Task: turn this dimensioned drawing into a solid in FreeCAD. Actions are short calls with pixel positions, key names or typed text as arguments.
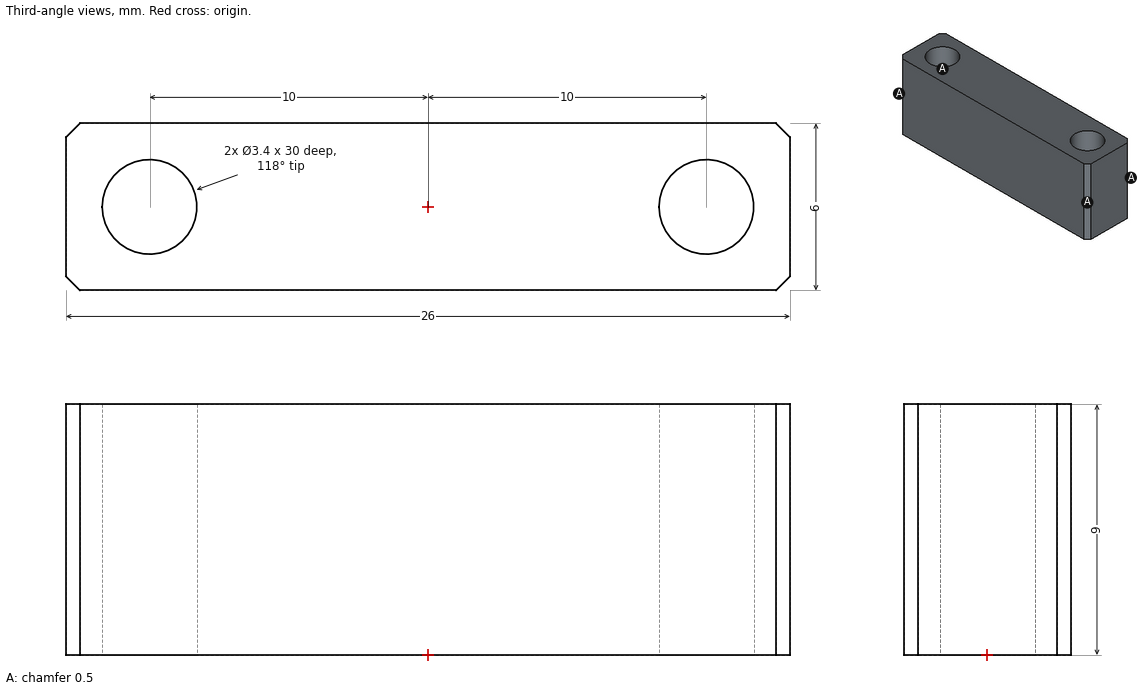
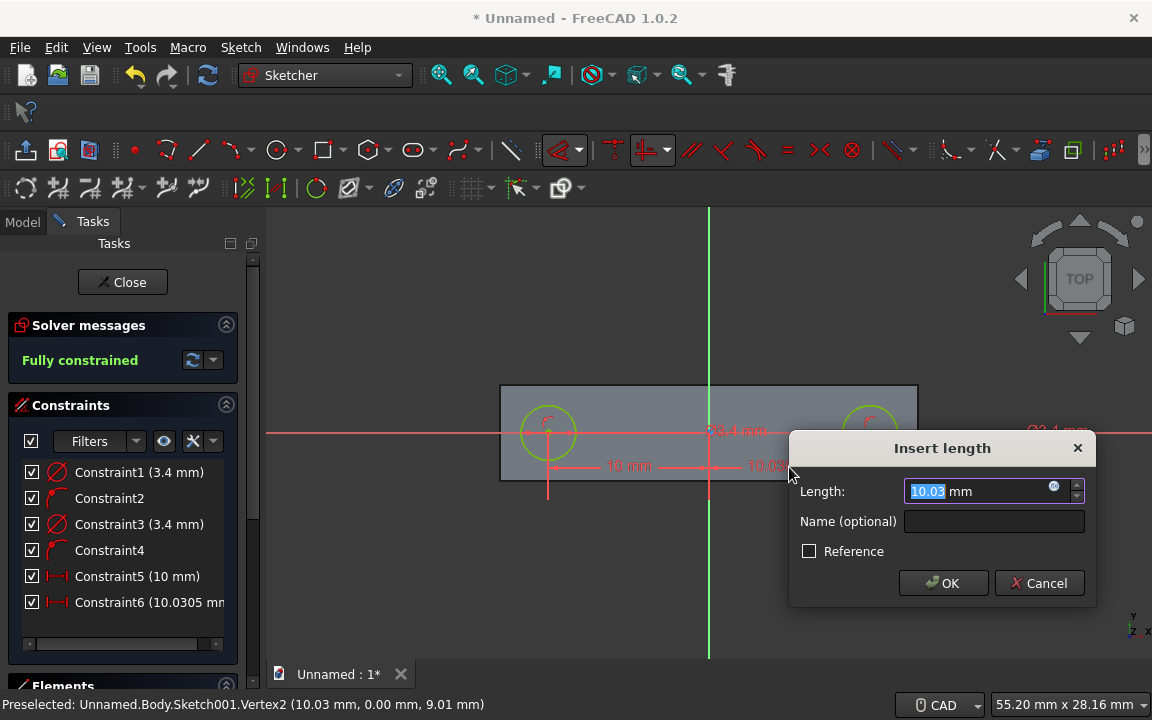
text(10)
key(Return)
key(Escape)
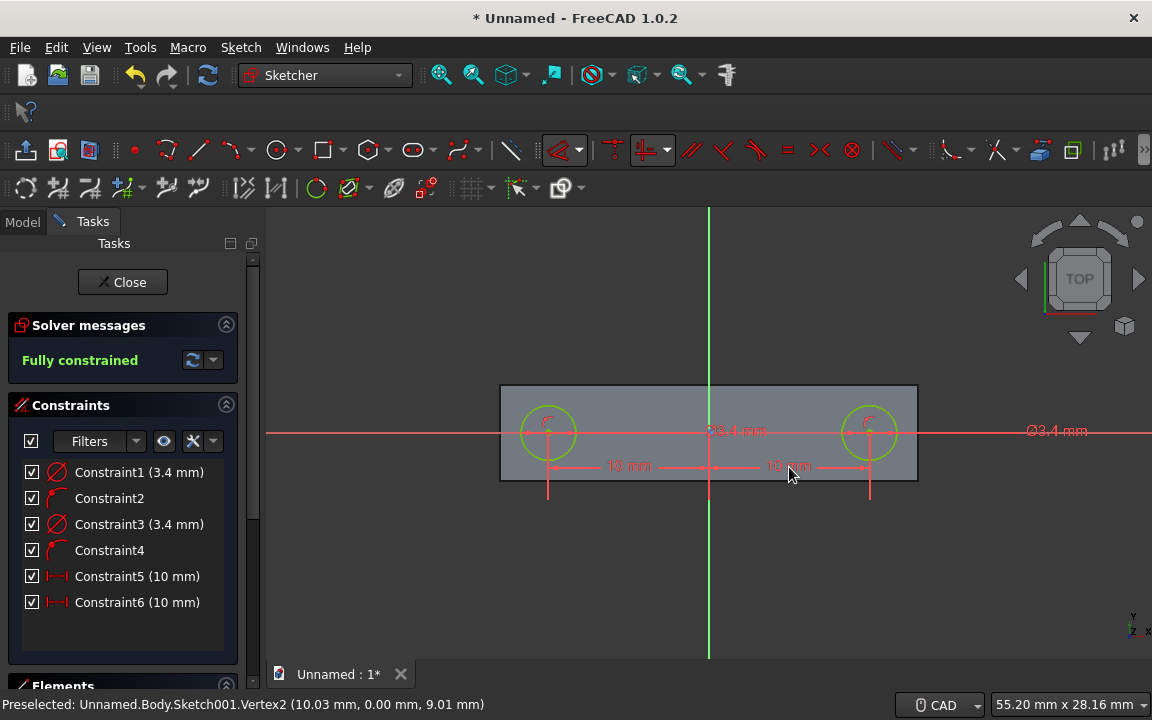
click(123, 282)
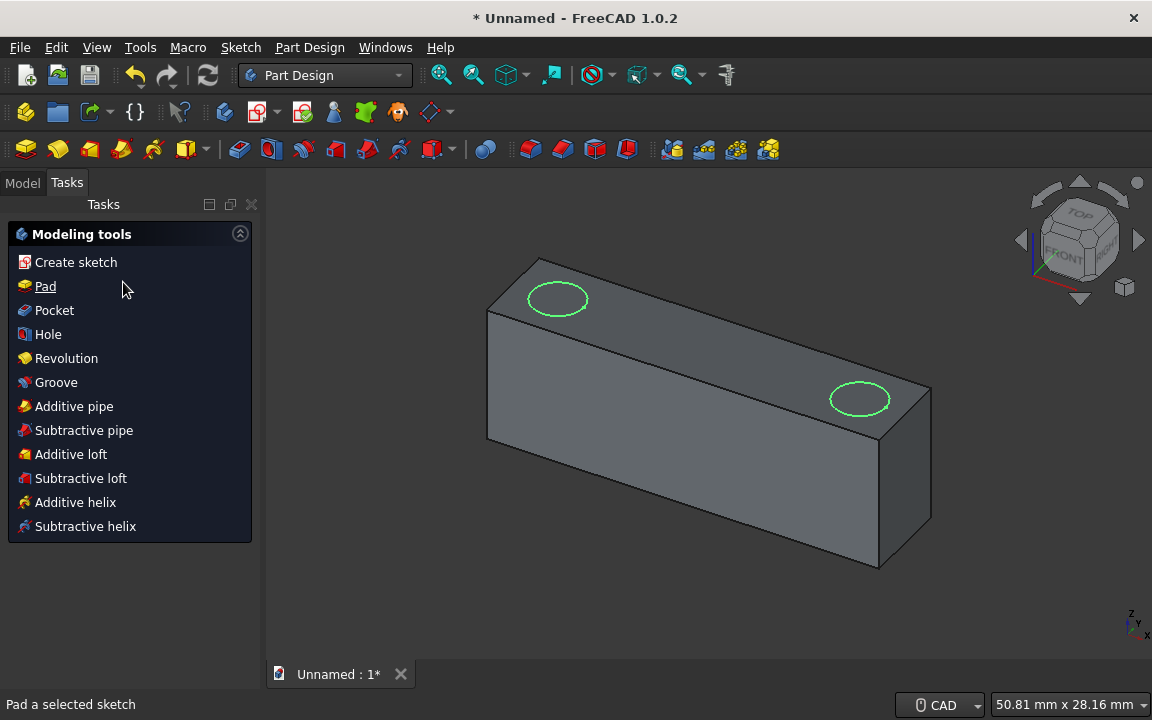
click(272, 150)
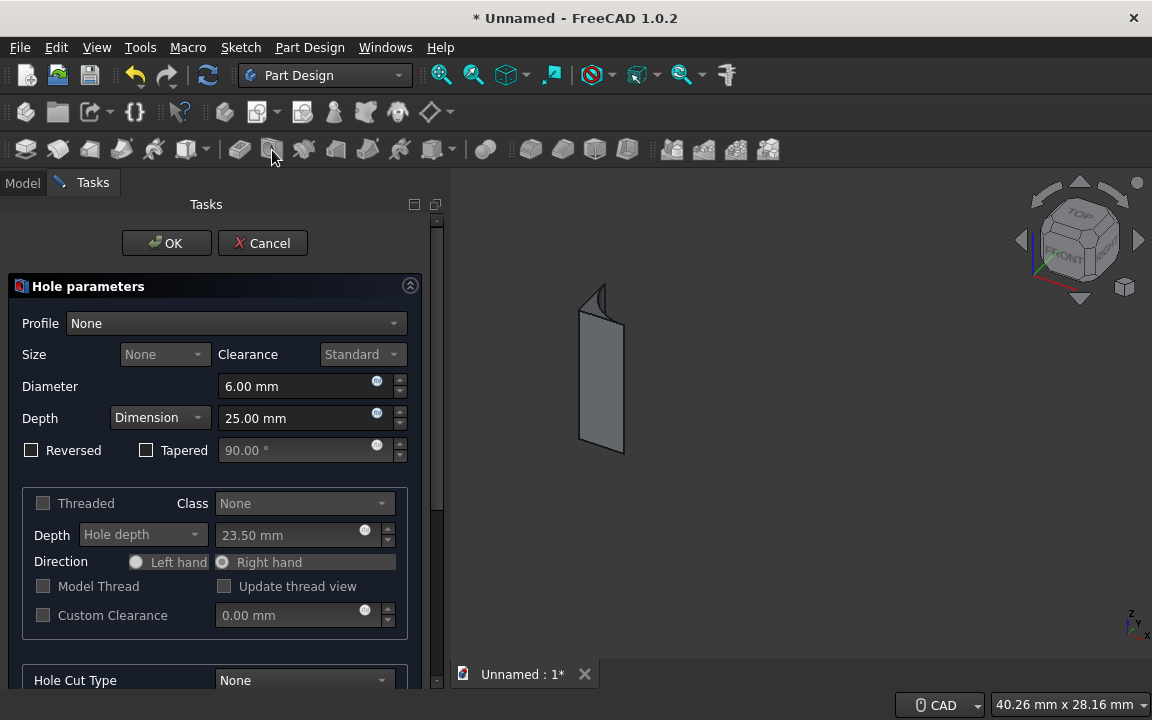
triple_click(305, 386)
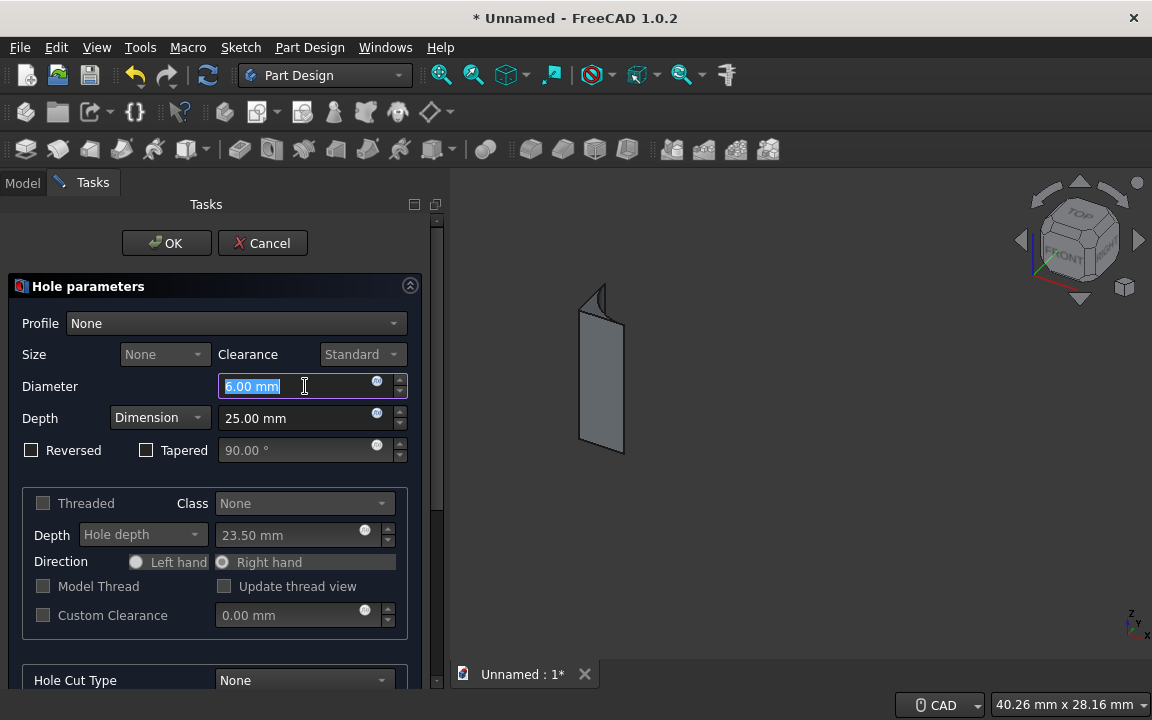
text(3.4)
key(Tab)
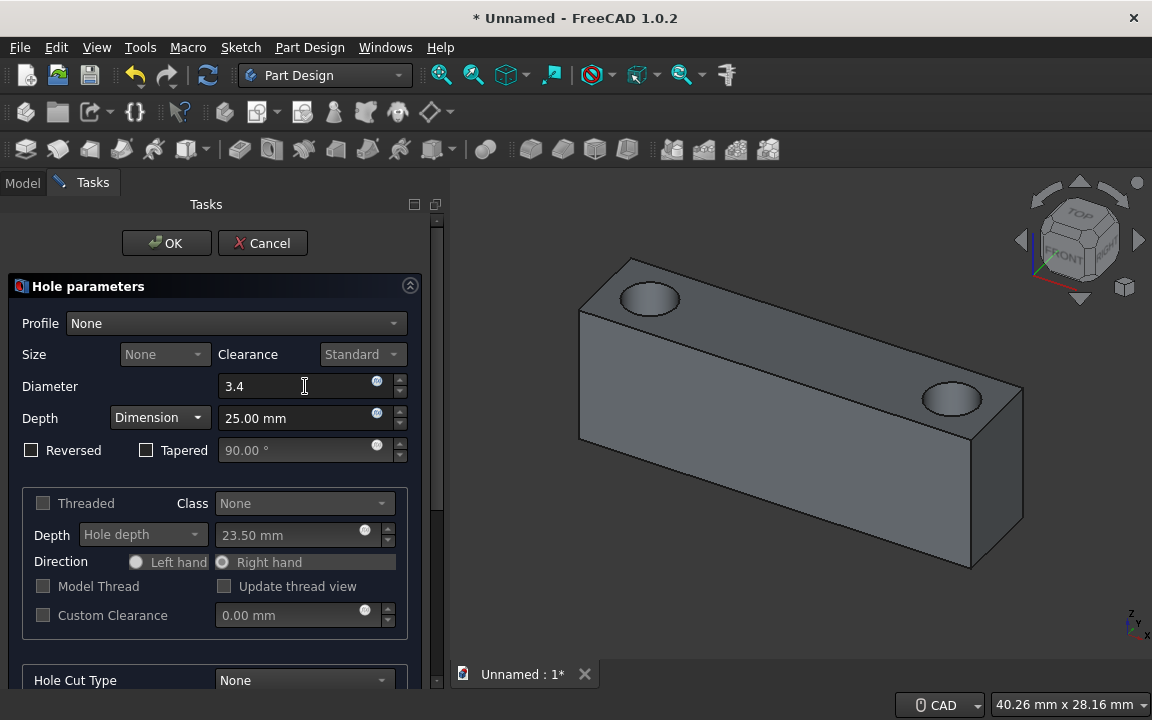
triple_click(305, 418)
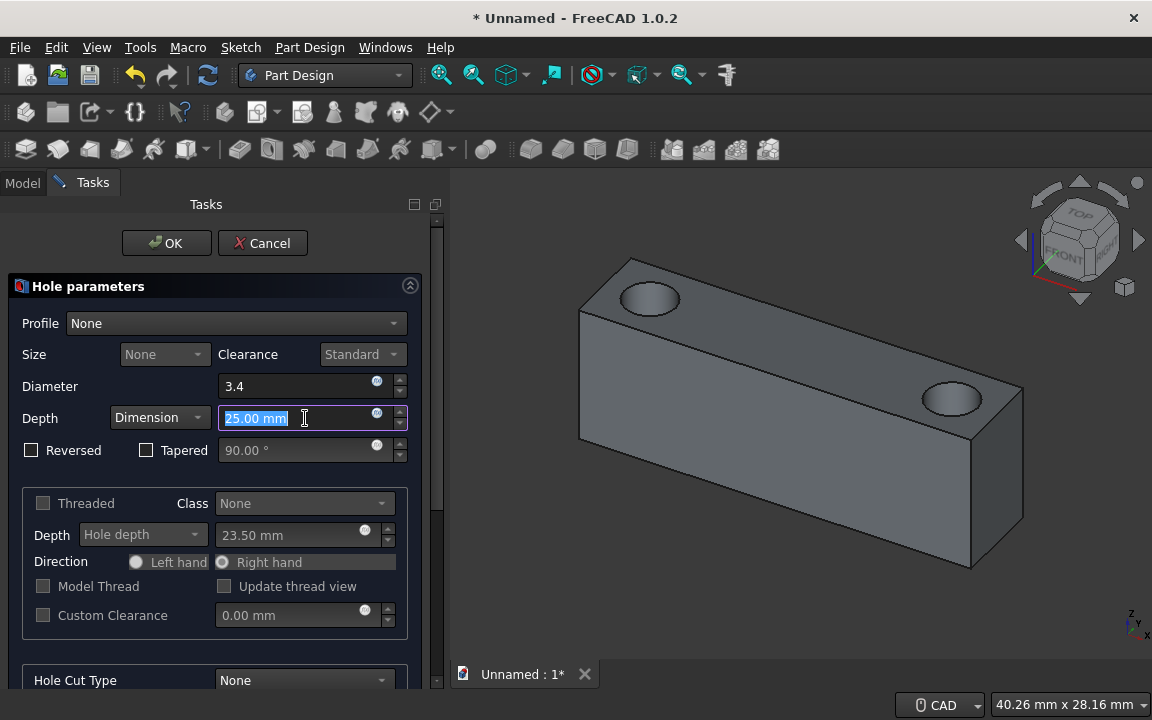
text(30)
key(Tab)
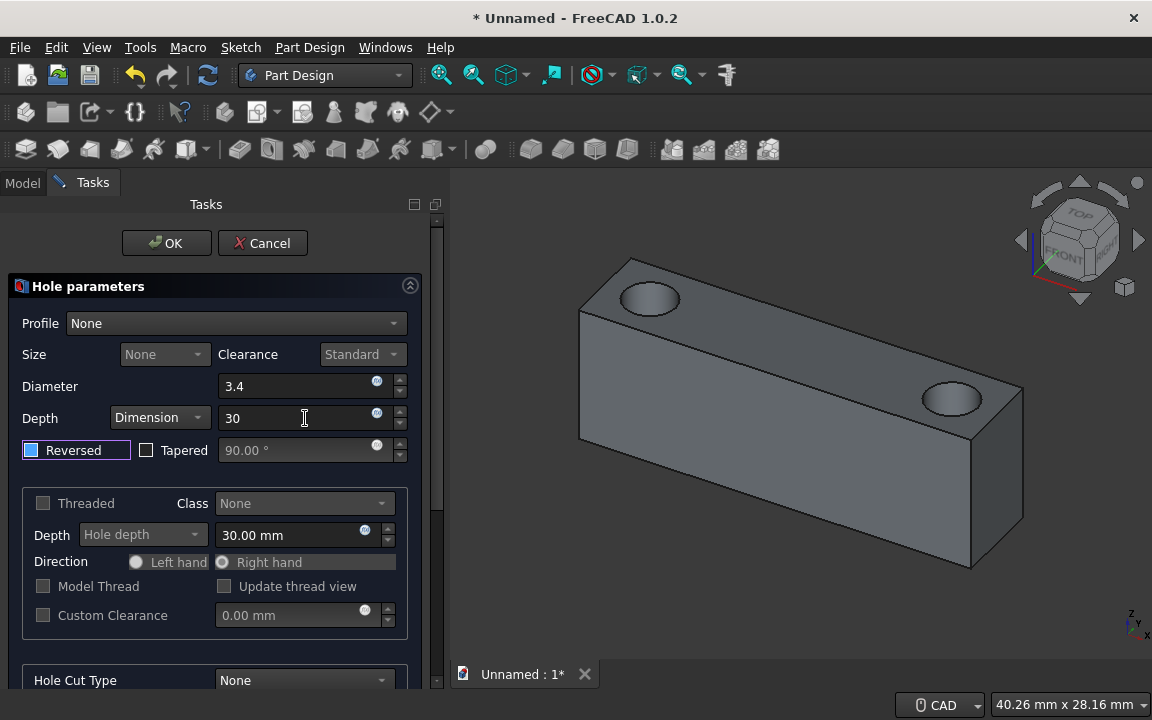
click(167, 243)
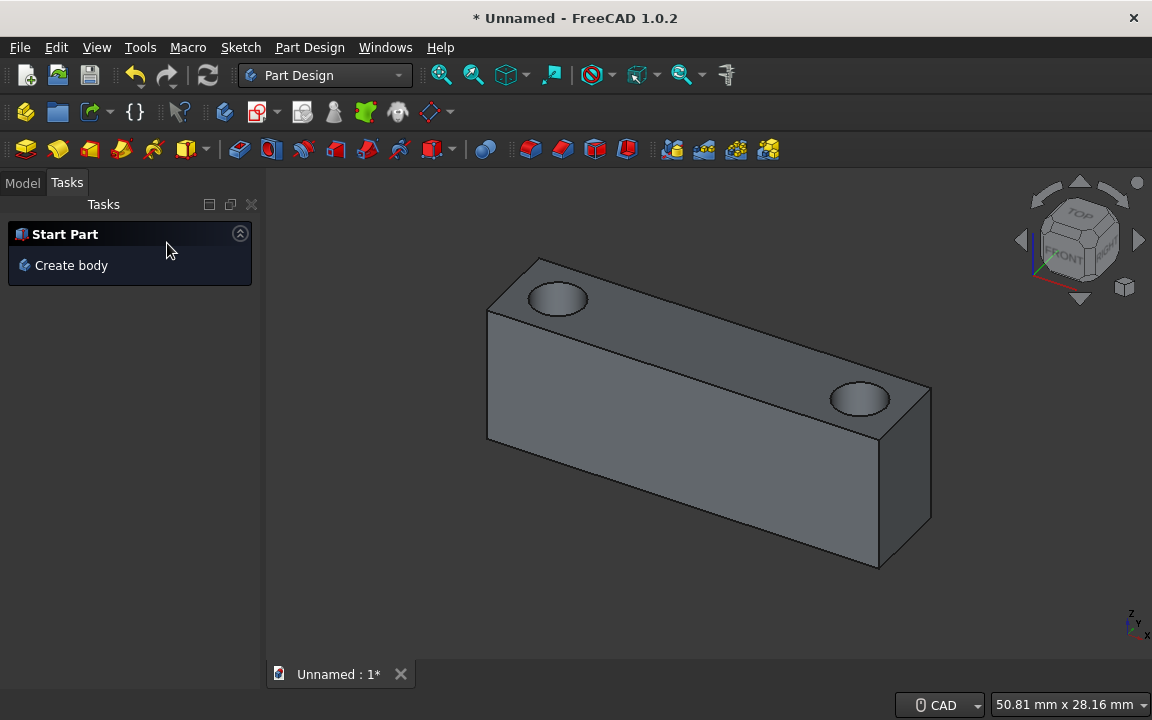
click(879, 503)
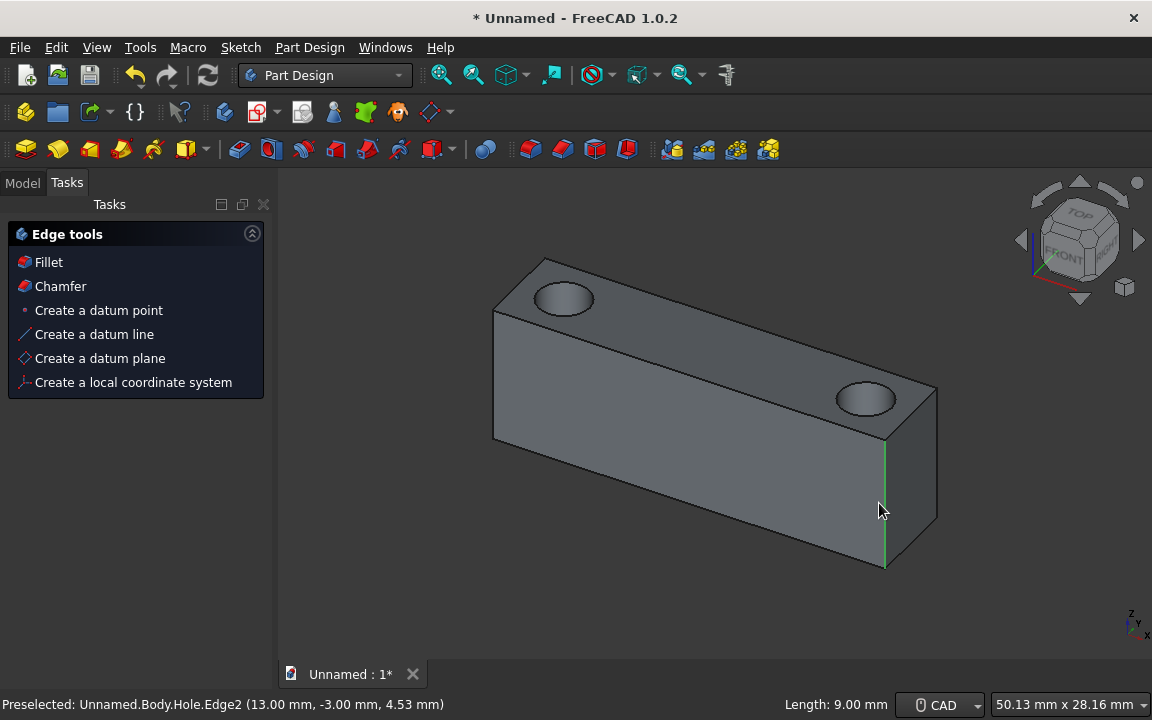
key(0)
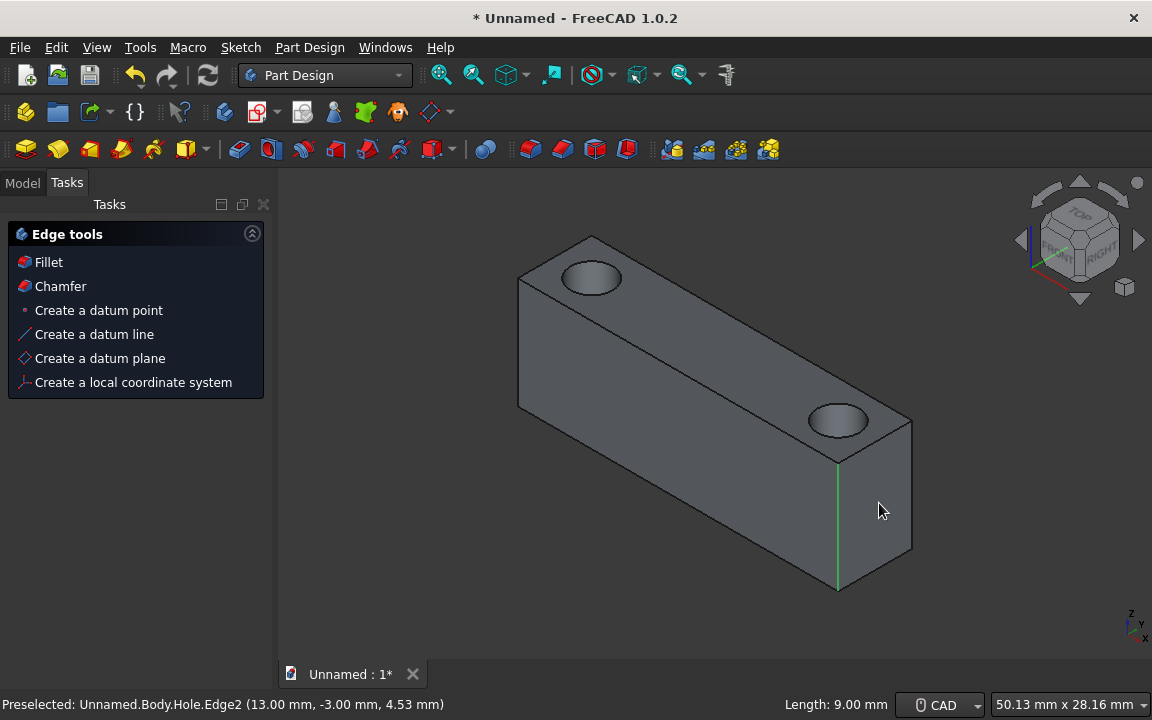
key(2)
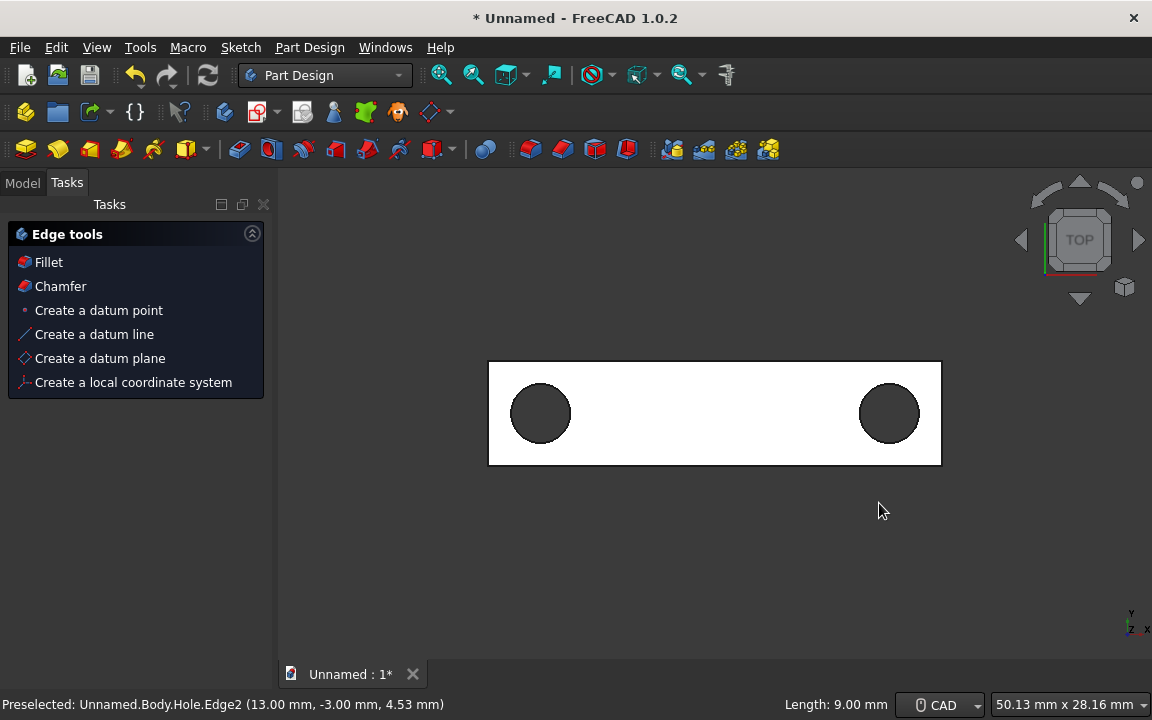
key(1)